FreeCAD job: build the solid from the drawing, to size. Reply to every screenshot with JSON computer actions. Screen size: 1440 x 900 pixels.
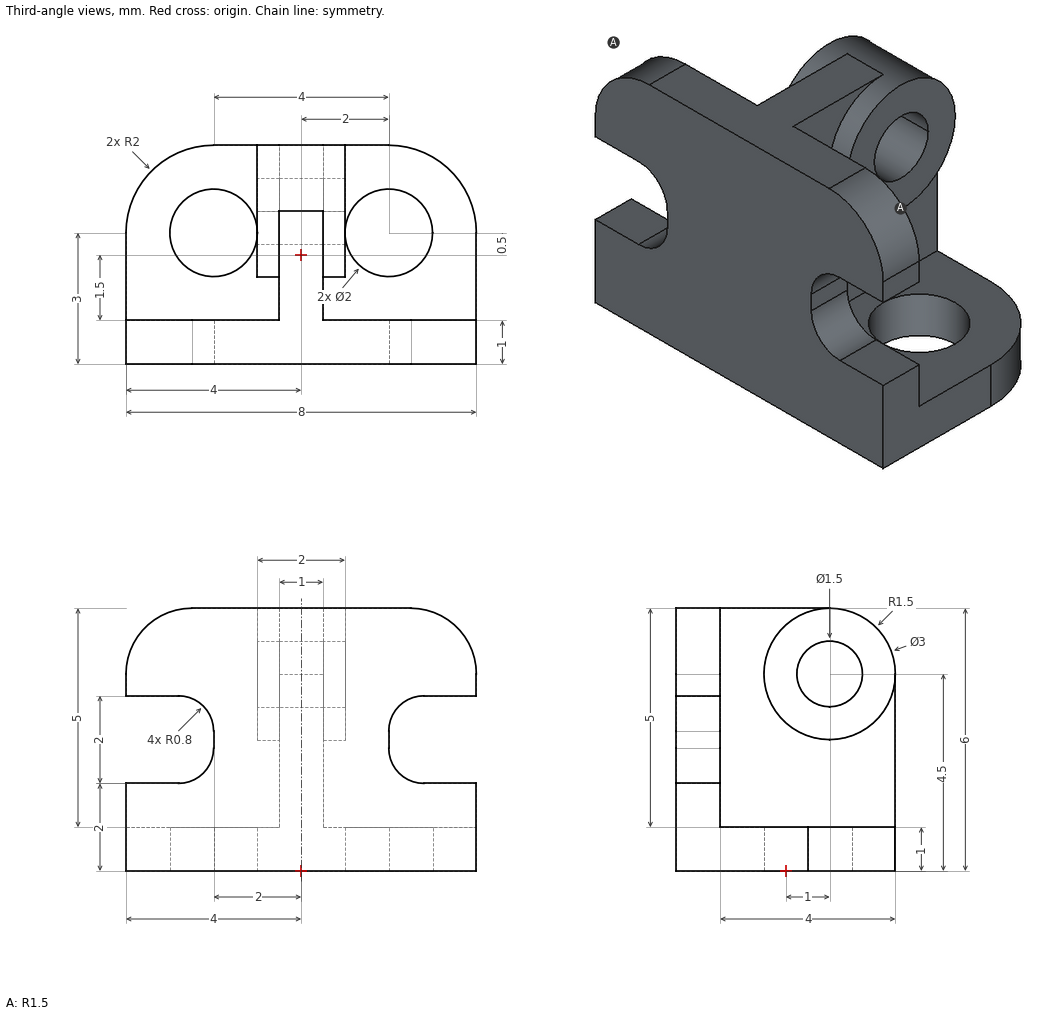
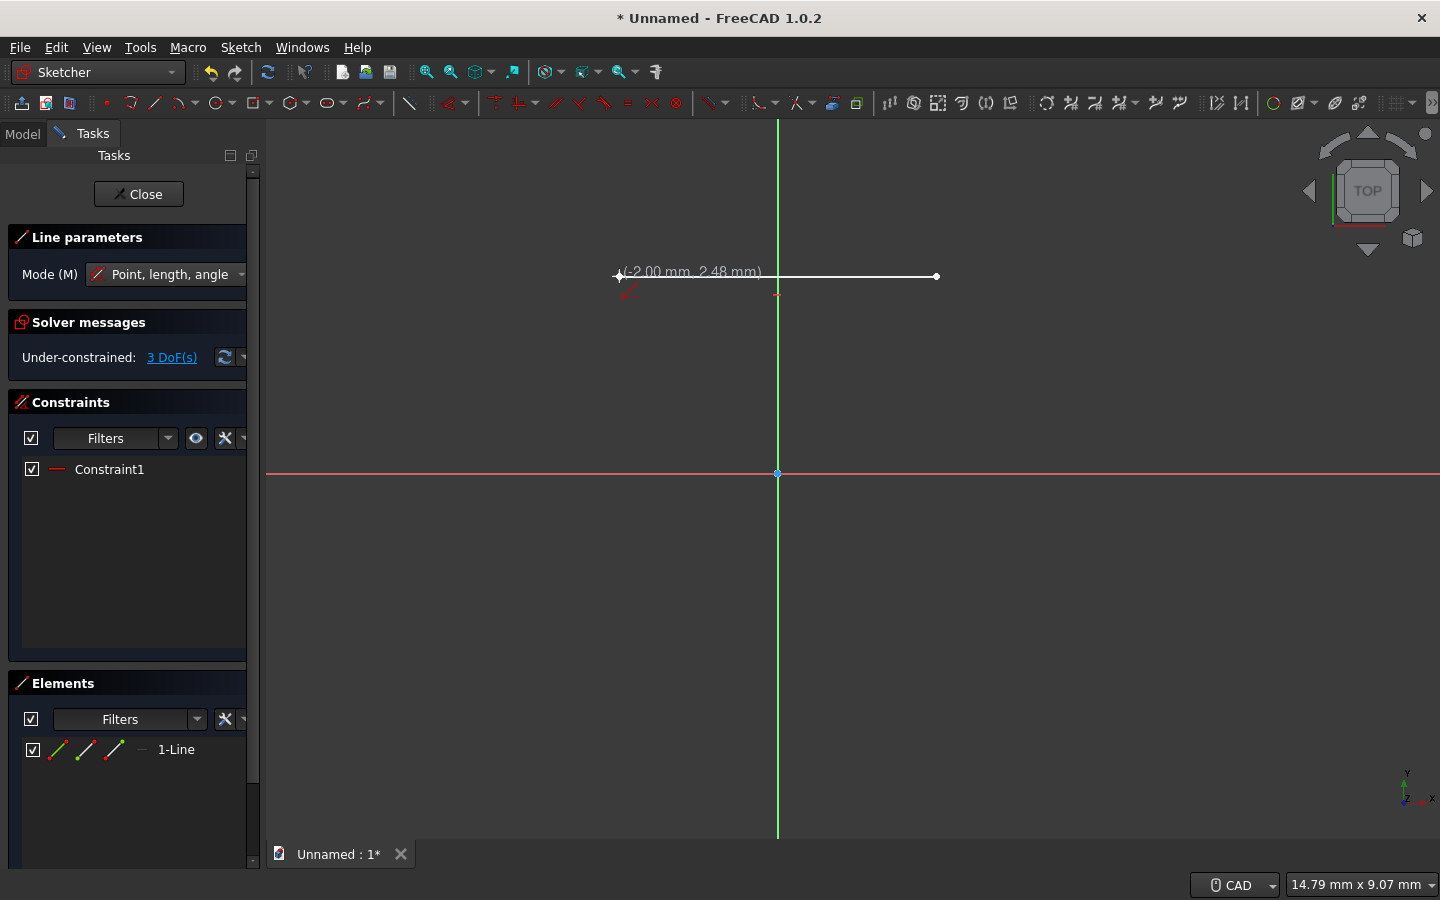
{"action": "left_click", "coordinate": [132, 104]}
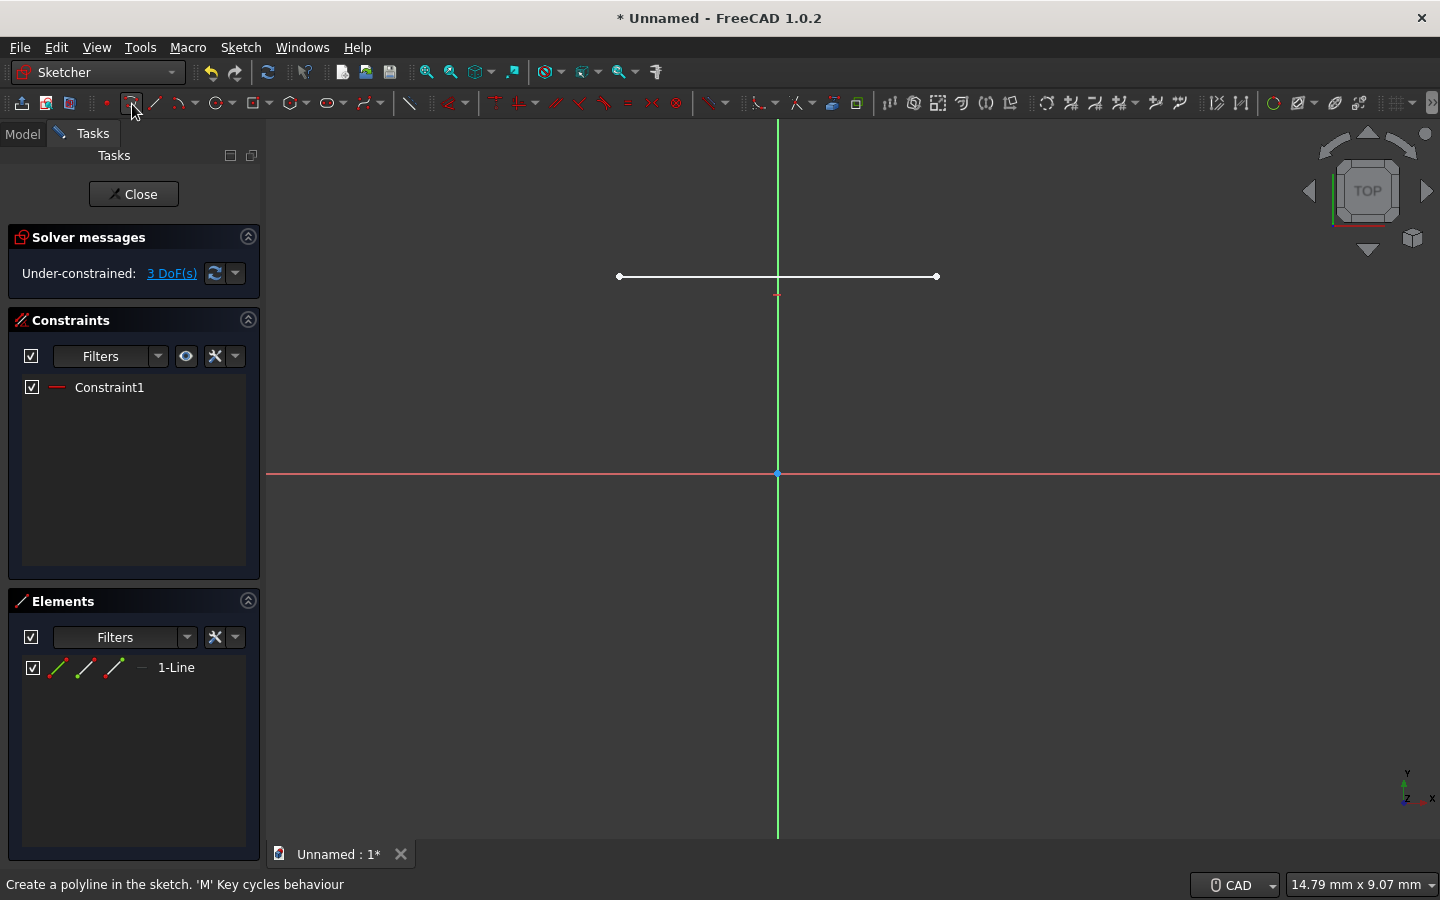
{"action": "left_click", "coordinate": [460, 434]}
{"action": "left_click", "coordinate": [460, 672]}
{"action": "left_click", "coordinate": [1095, 672]}
{"action": "left_click", "coordinate": [1095, 434]}
{"action": "right_click", "coordinate": [1095, 434]}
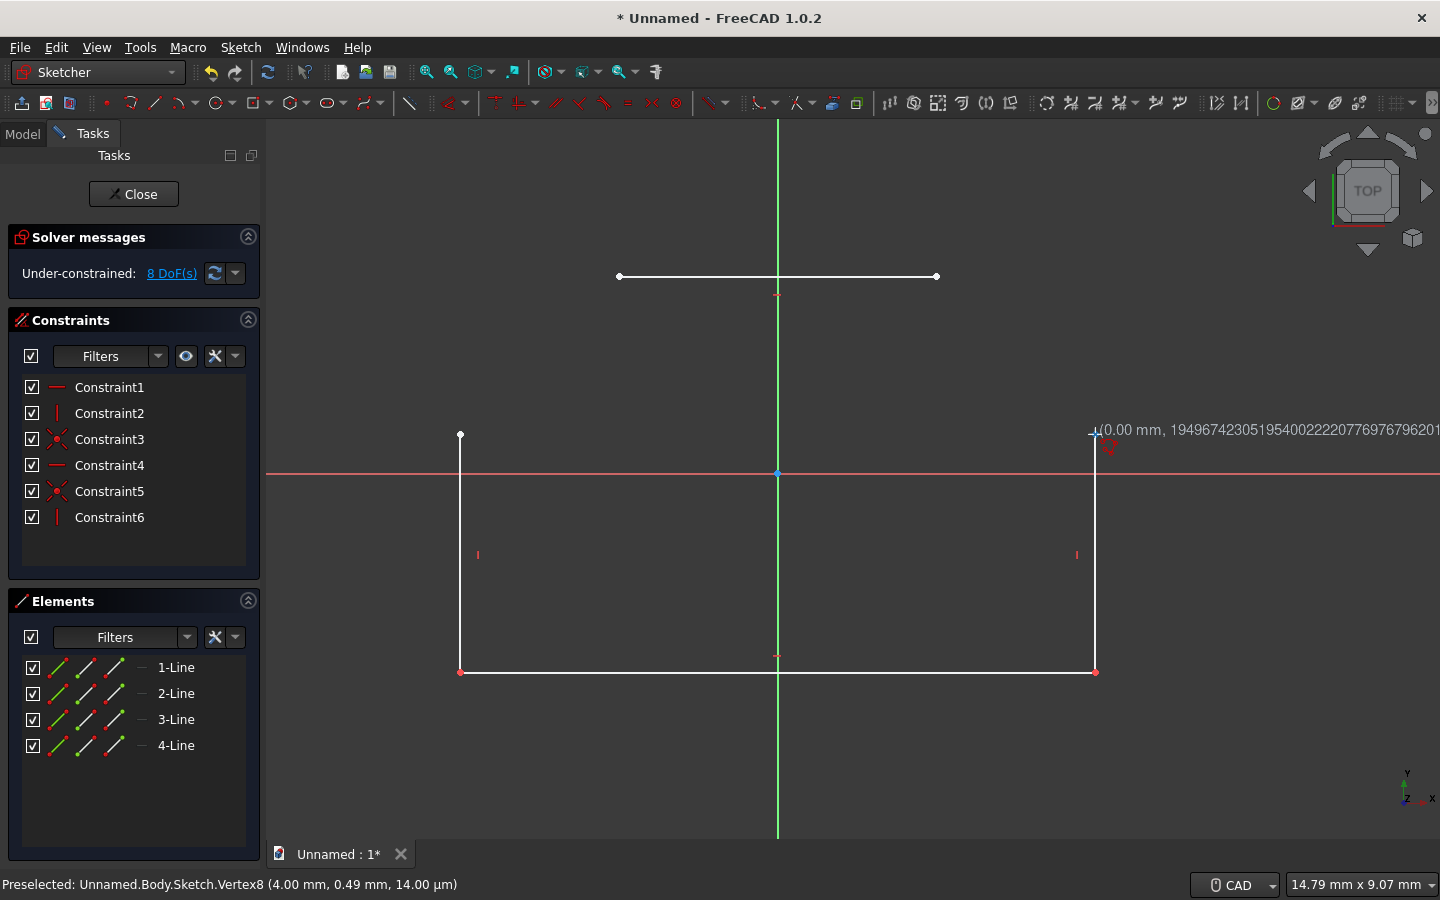
{"action": "left_click", "coordinate": [198, 104]}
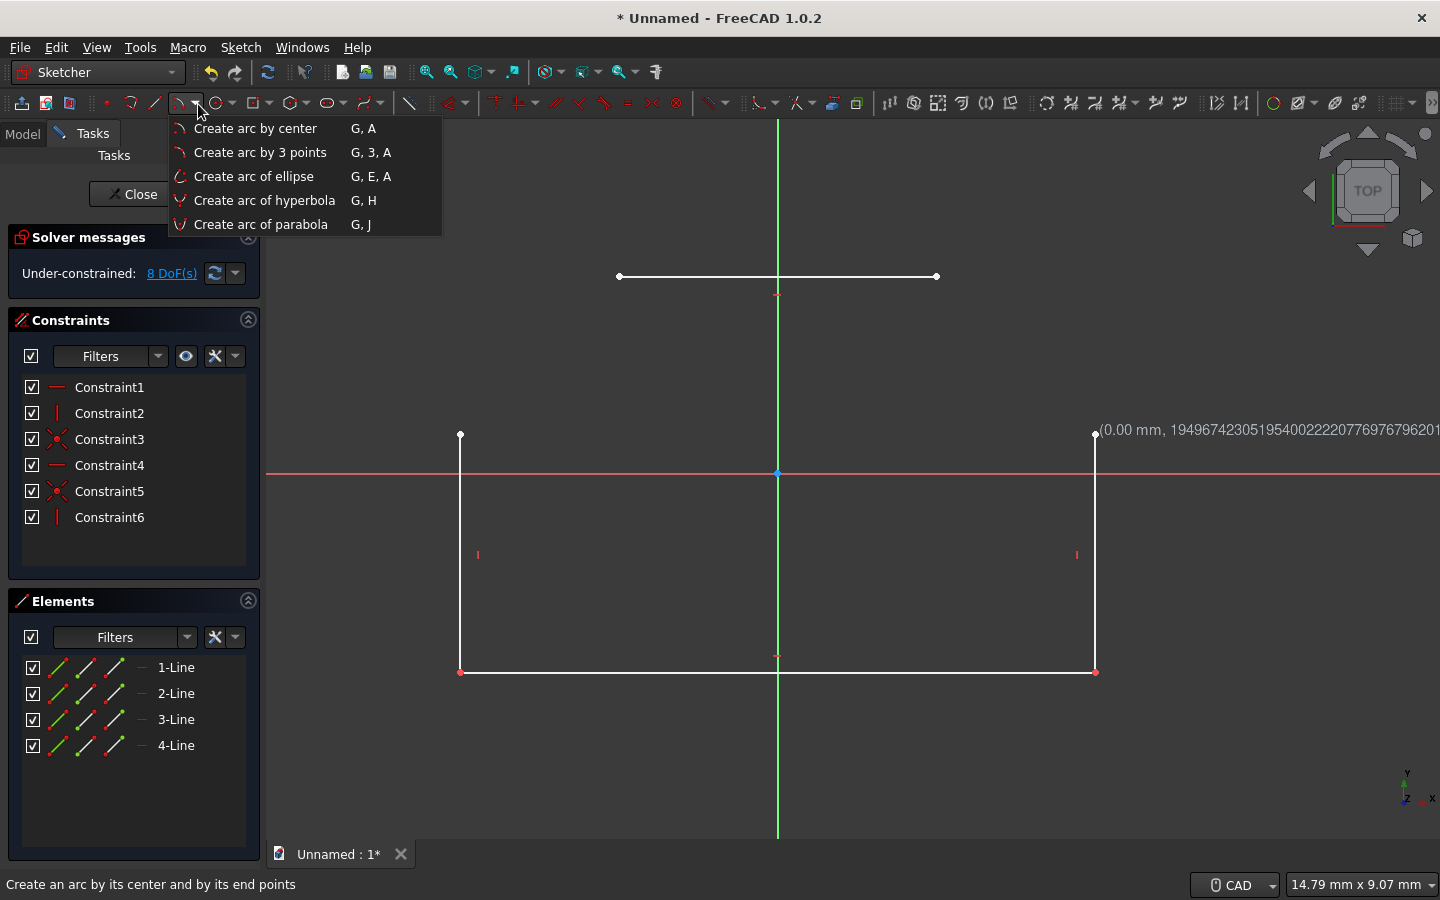
{"action": "left_click", "coordinate": [306, 152]}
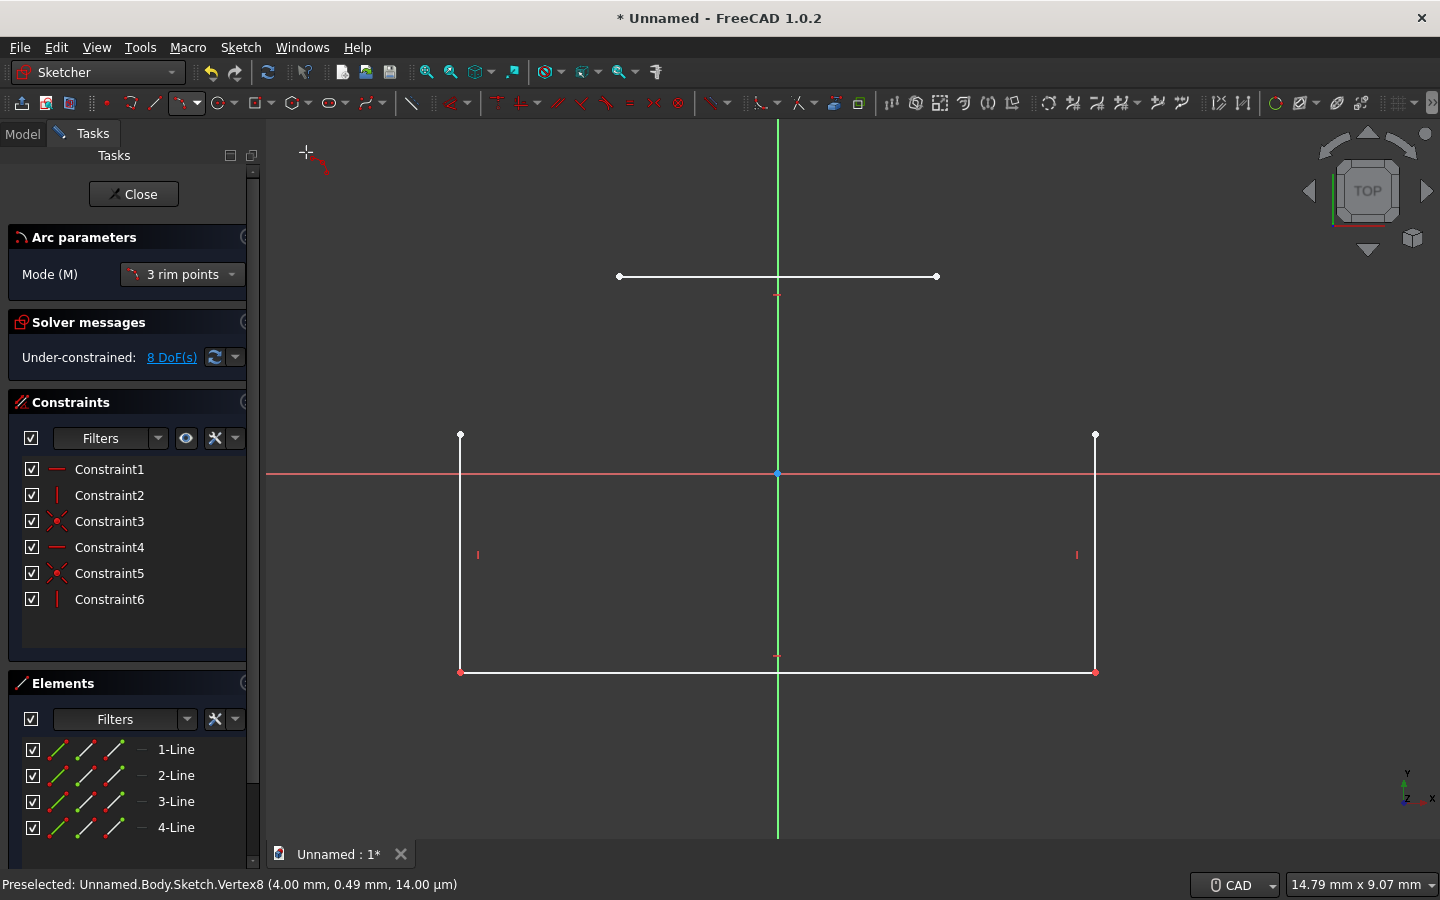
{"action": "left_click", "coordinate": [619, 277]}
{"action": "left_click", "coordinate": [460, 435]}
{"action": "left_click", "coordinate": [507, 322]}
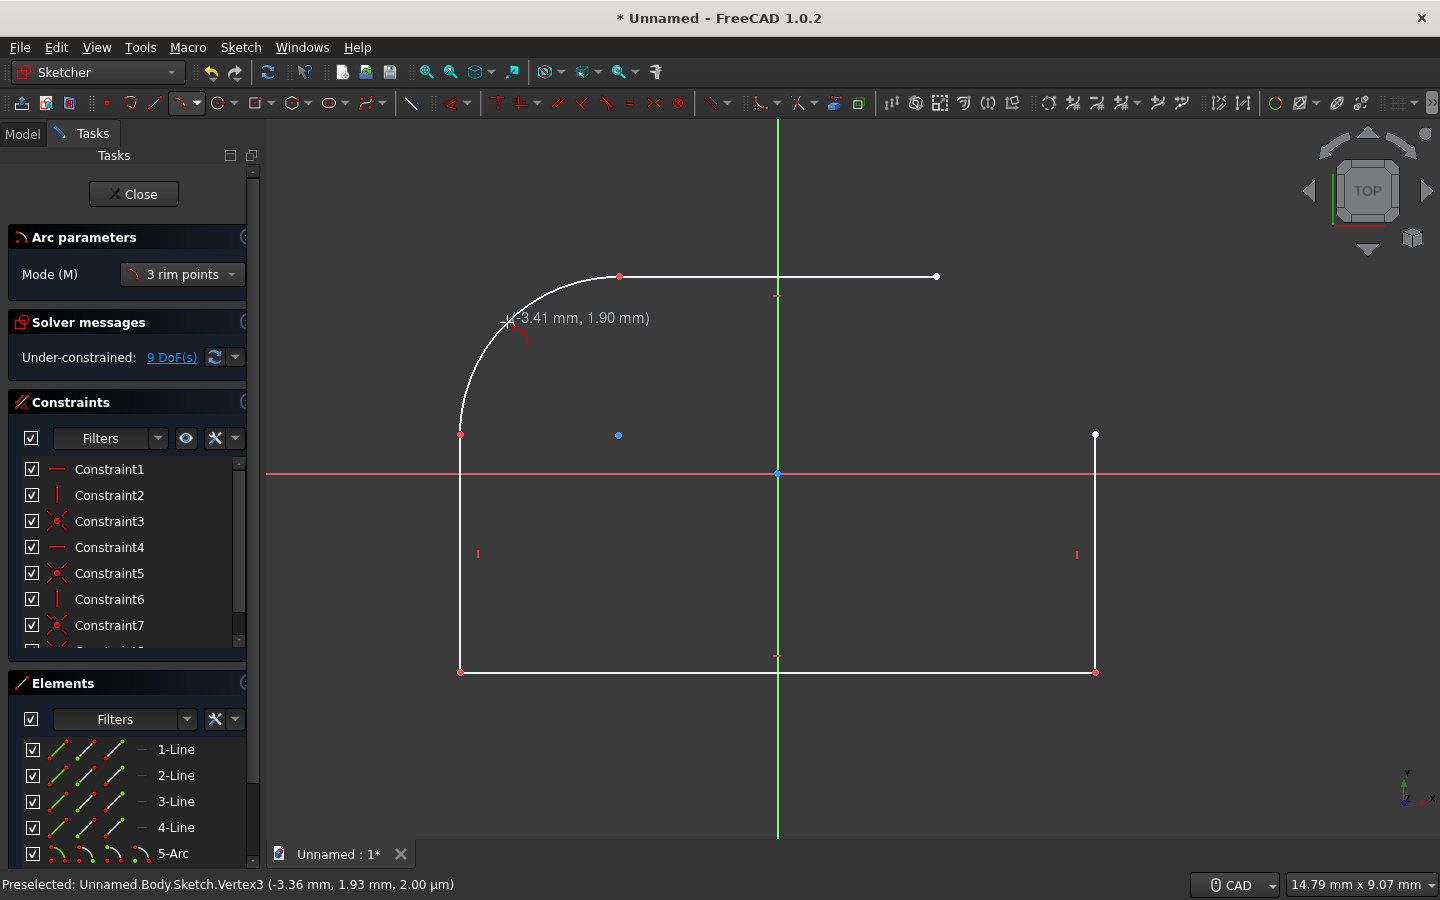
{"action": "left_click", "coordinate": [1095, 435]}
{"action": "left_click", "coordinate": [936, 277]}
{"action": "left_click", "coordinate": [1049, 322]}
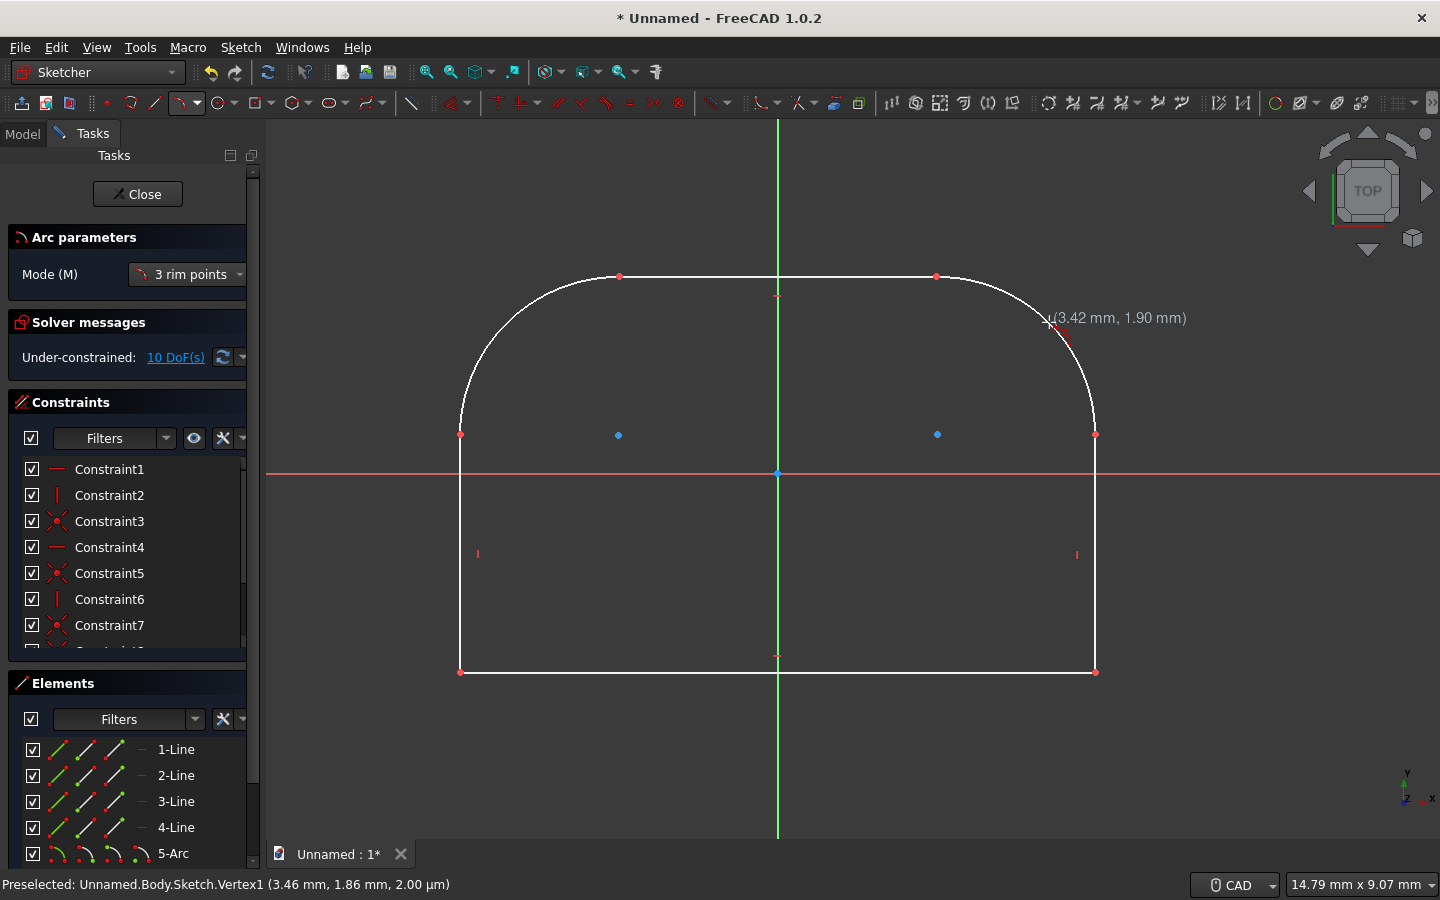
{"action": "left_click", "coordinate": [218, 104]}